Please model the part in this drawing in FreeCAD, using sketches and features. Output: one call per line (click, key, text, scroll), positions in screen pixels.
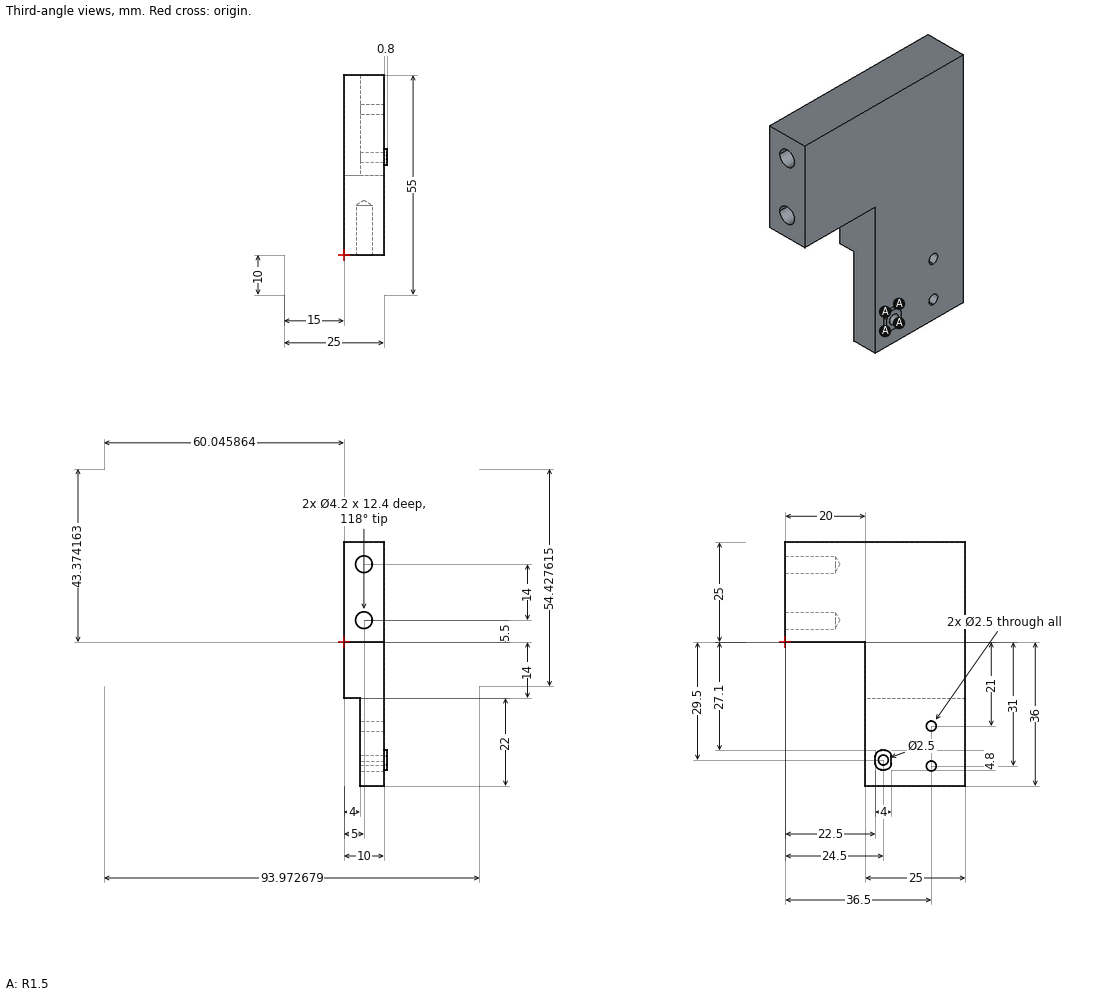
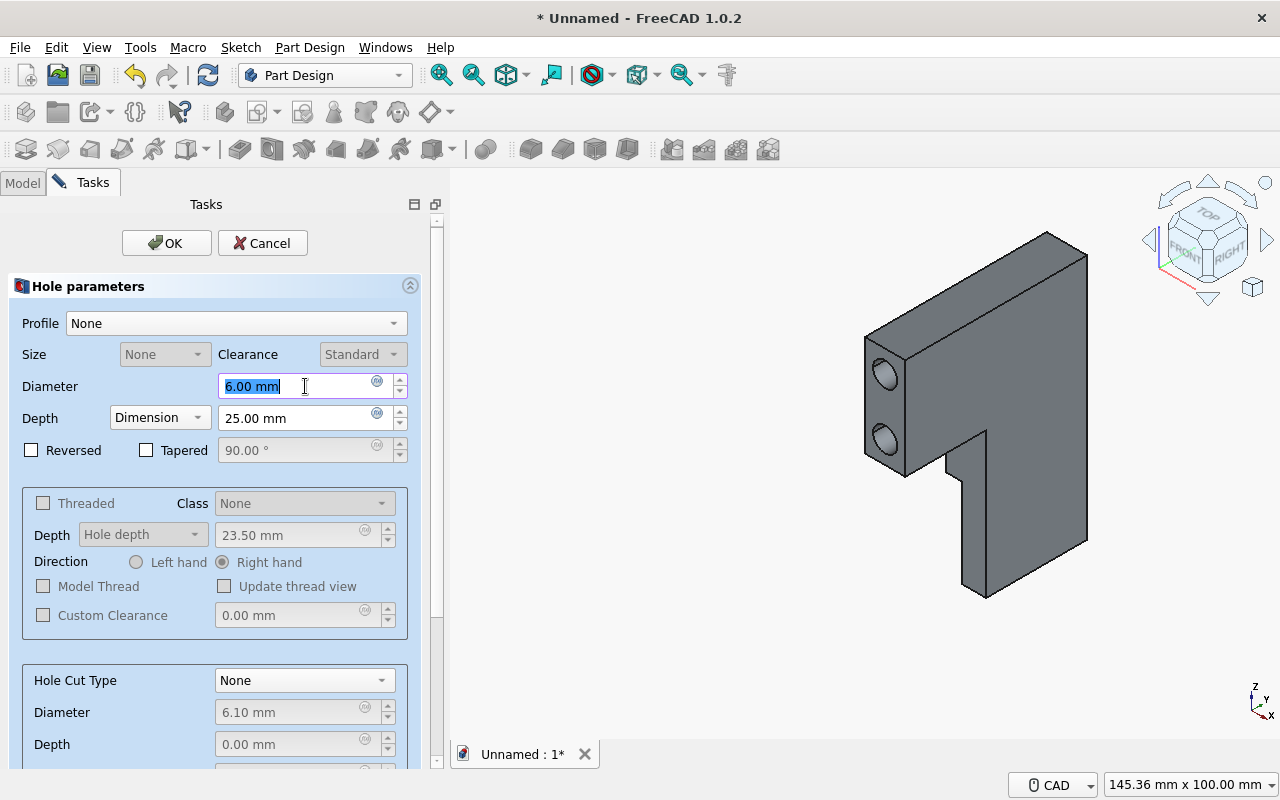
text(4.2)
key(Tab)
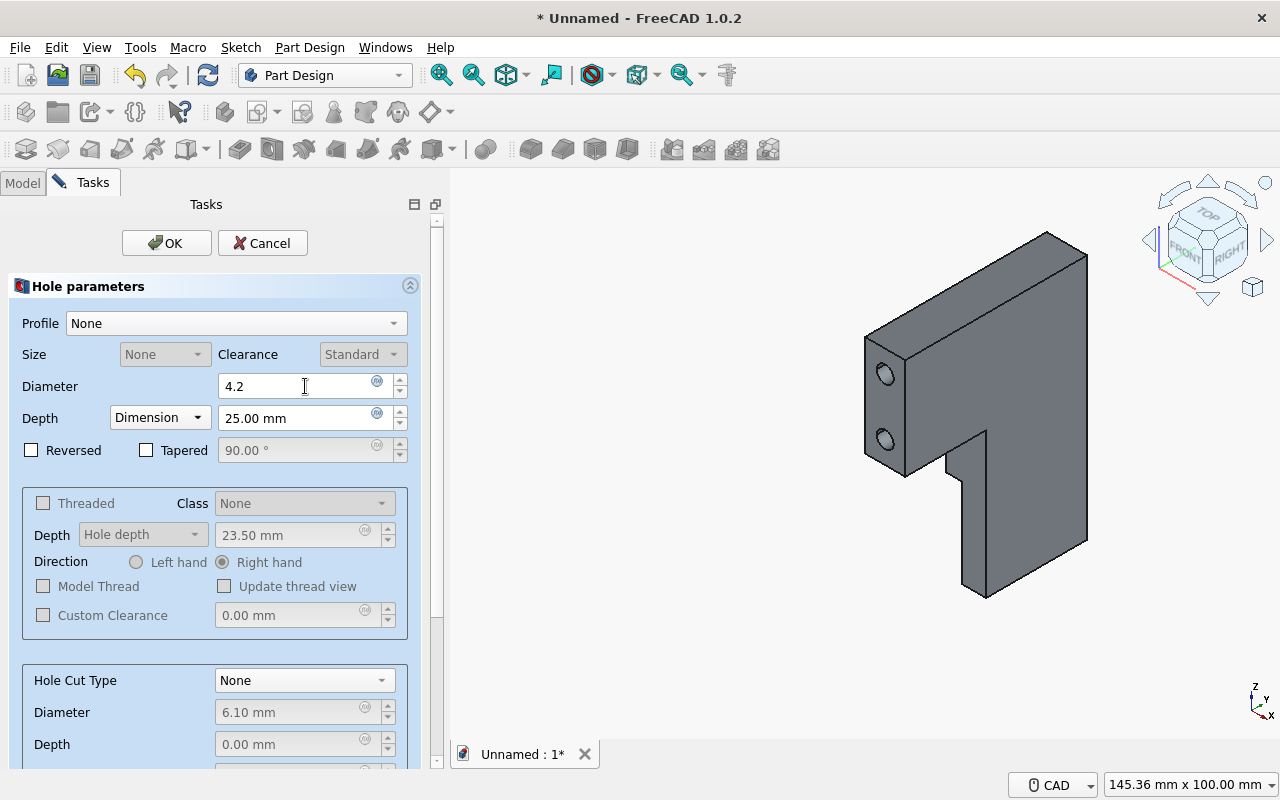
triple_click(305, 418)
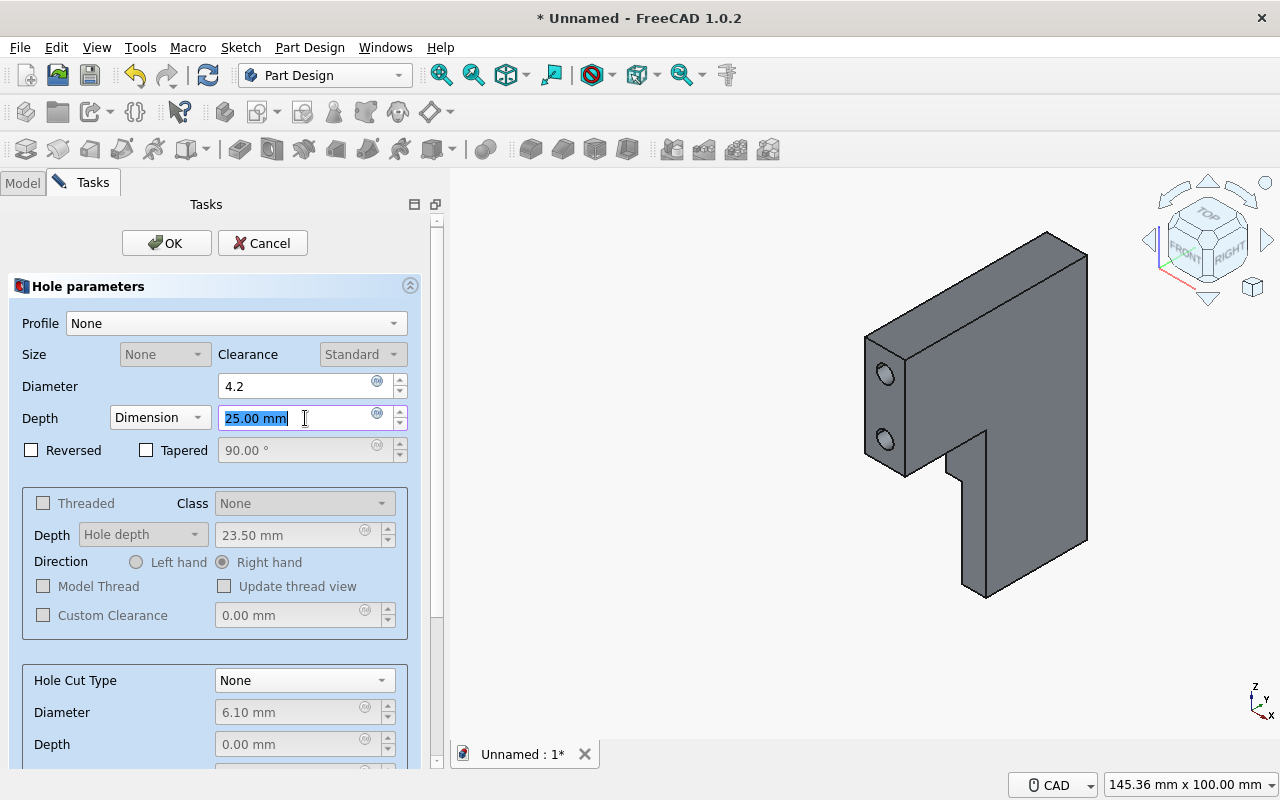
text(12.4)
key(Tab)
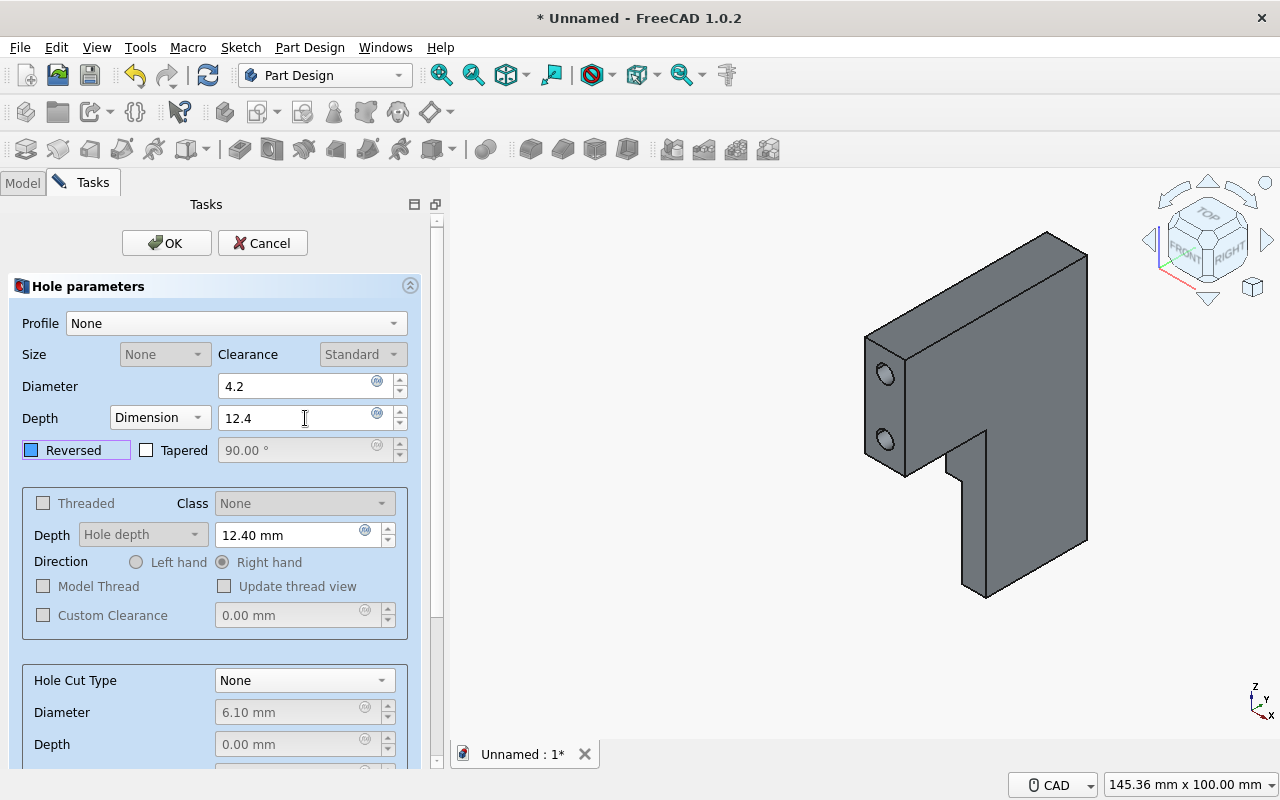
click(167, 243)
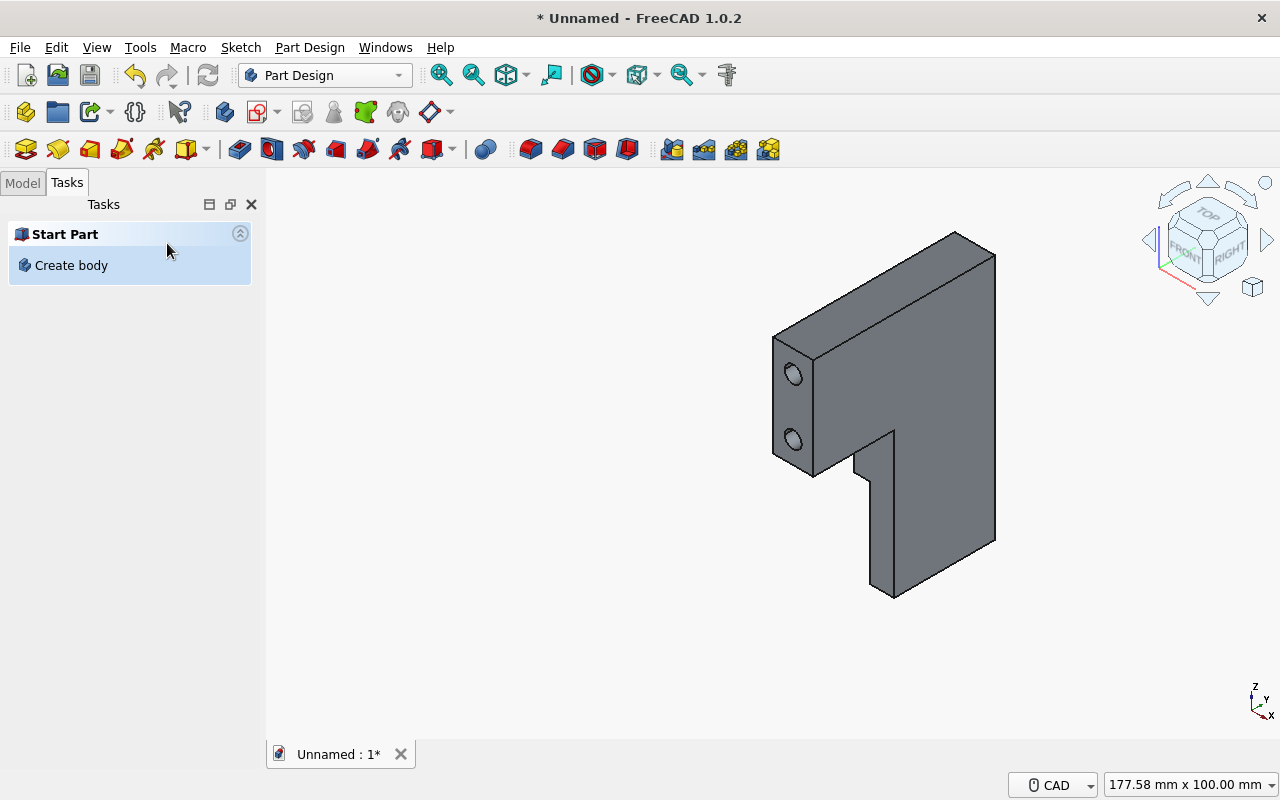
click(930, 353)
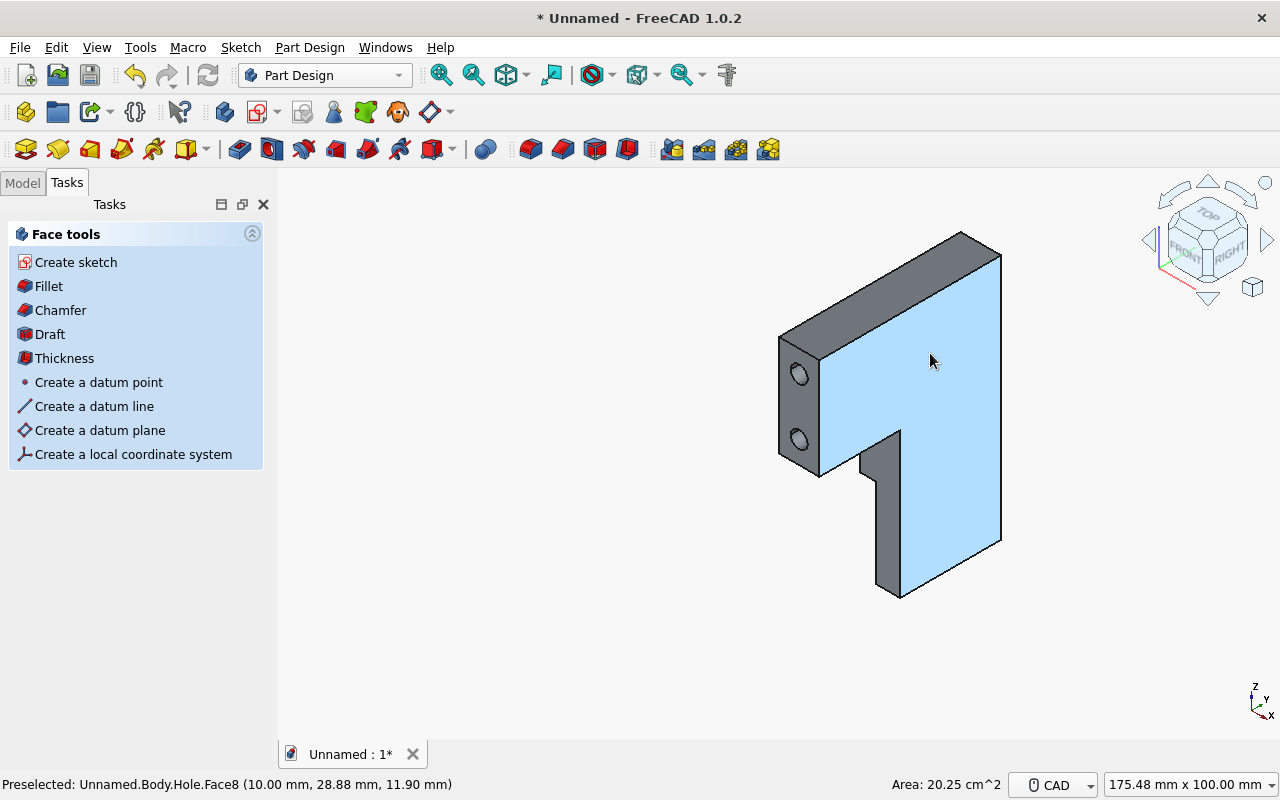
click(258, 112)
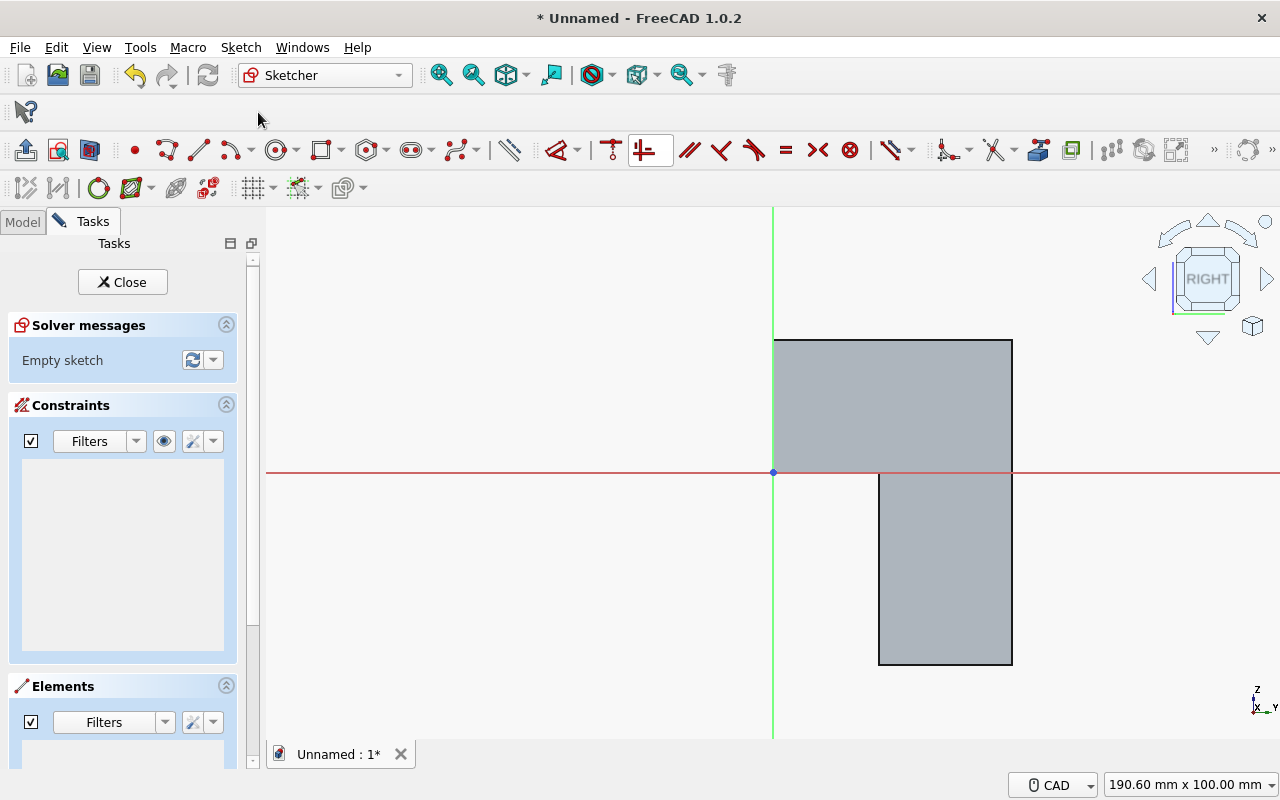
scroll(1034, 646, up, 8)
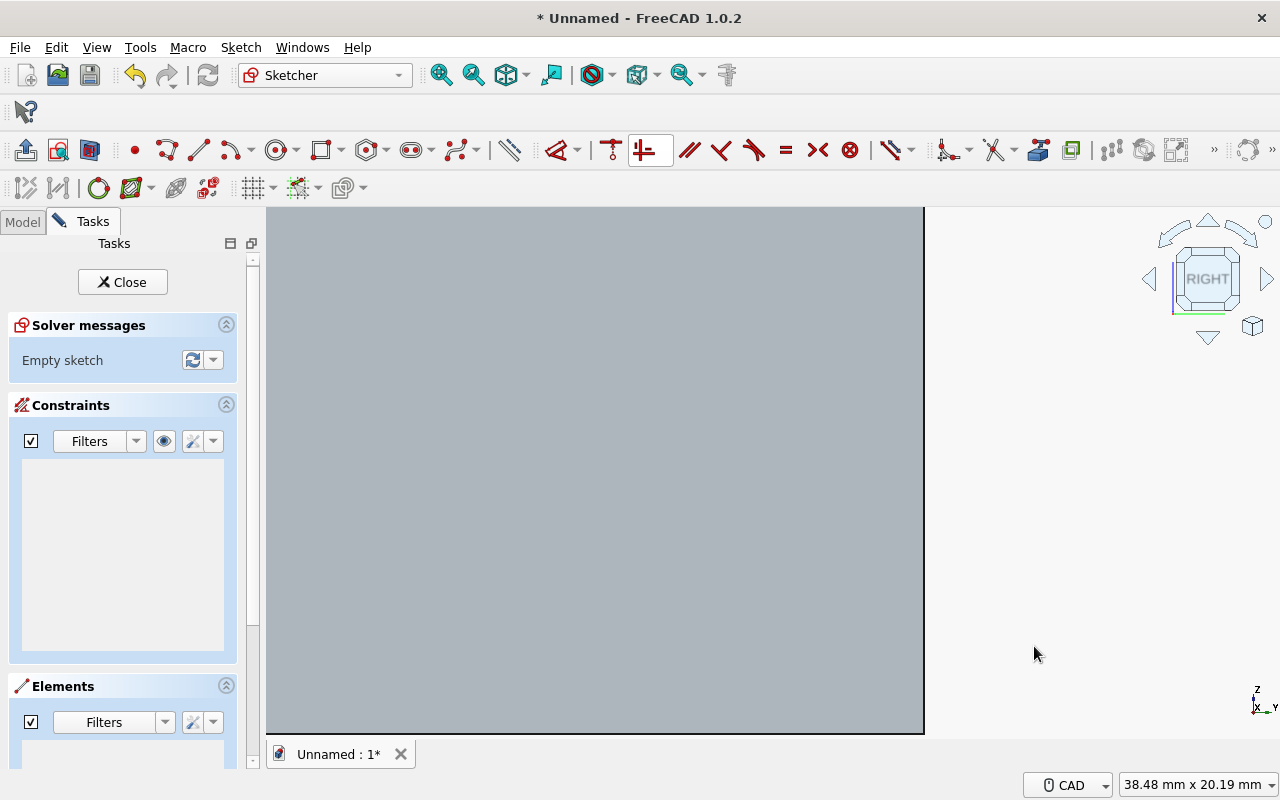
click(276, 150)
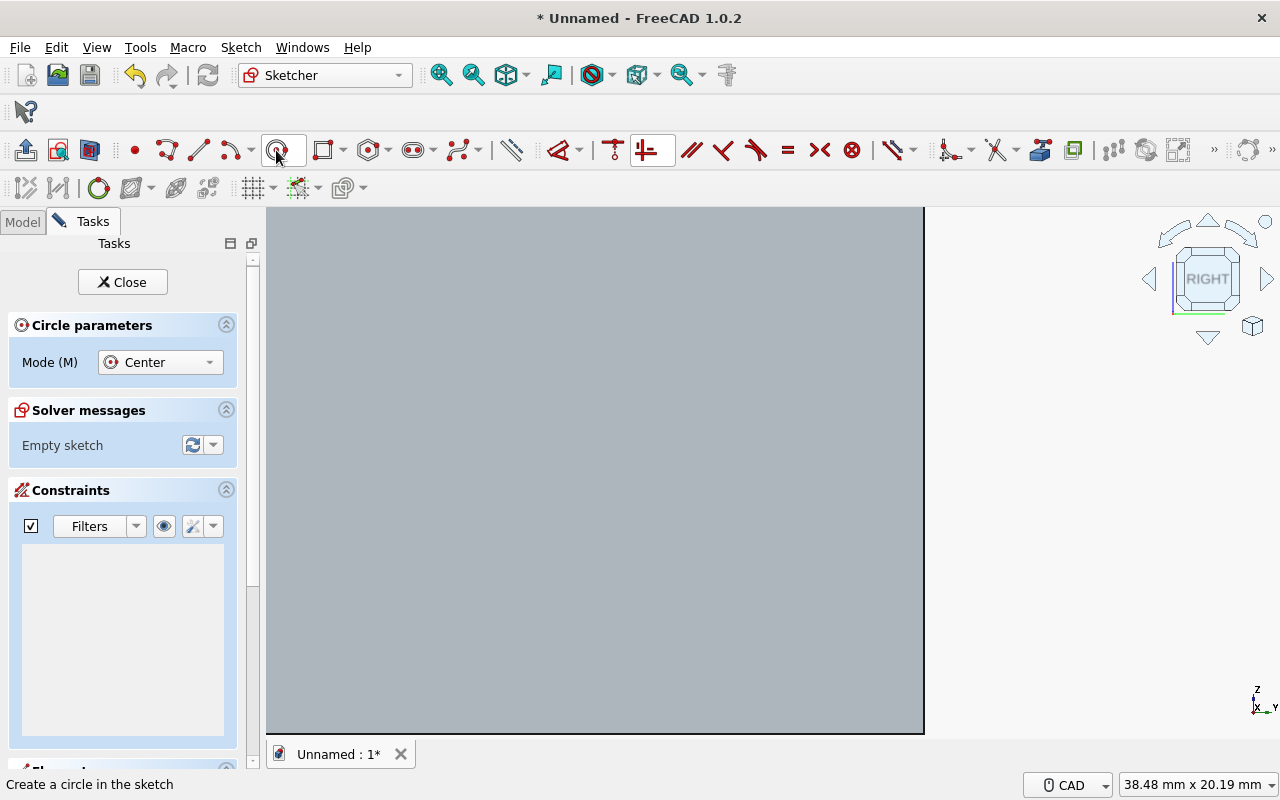
click(700, 339)
move(723, 316)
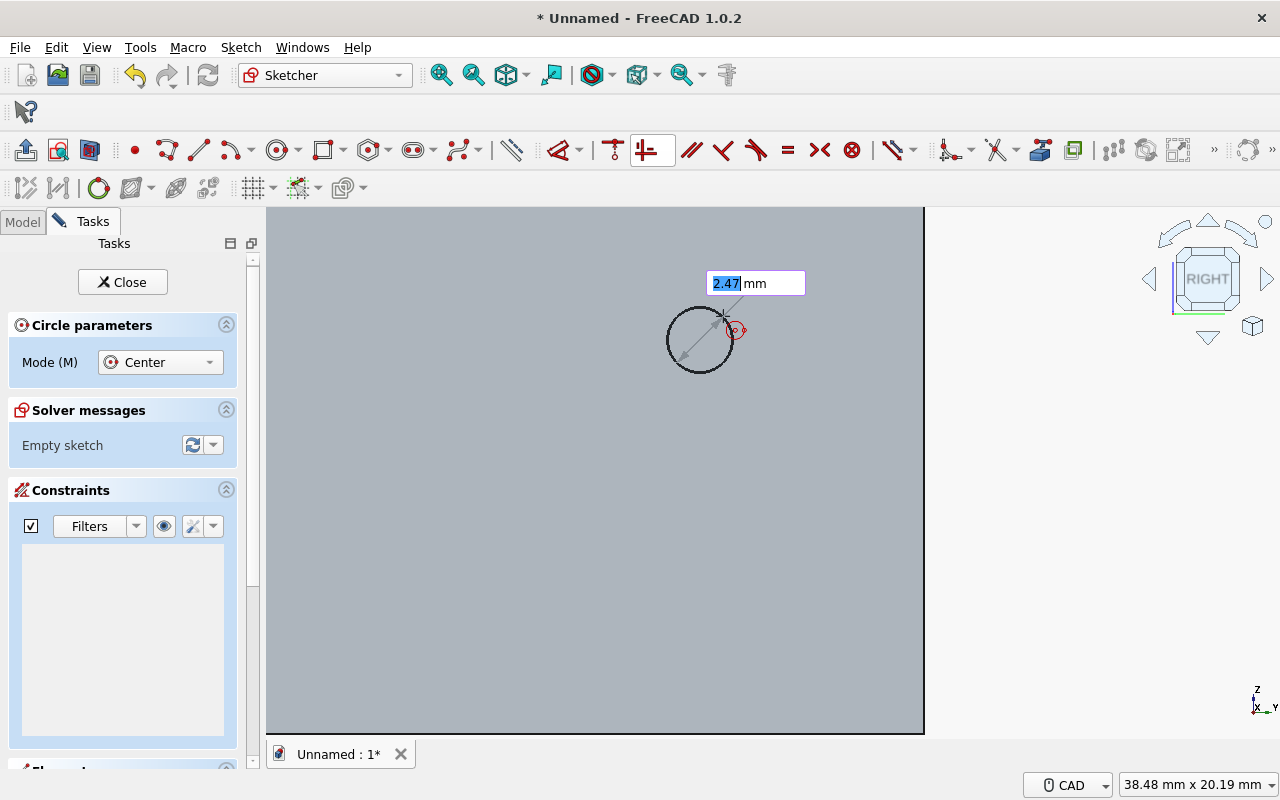
text(2.5)
key(Return)